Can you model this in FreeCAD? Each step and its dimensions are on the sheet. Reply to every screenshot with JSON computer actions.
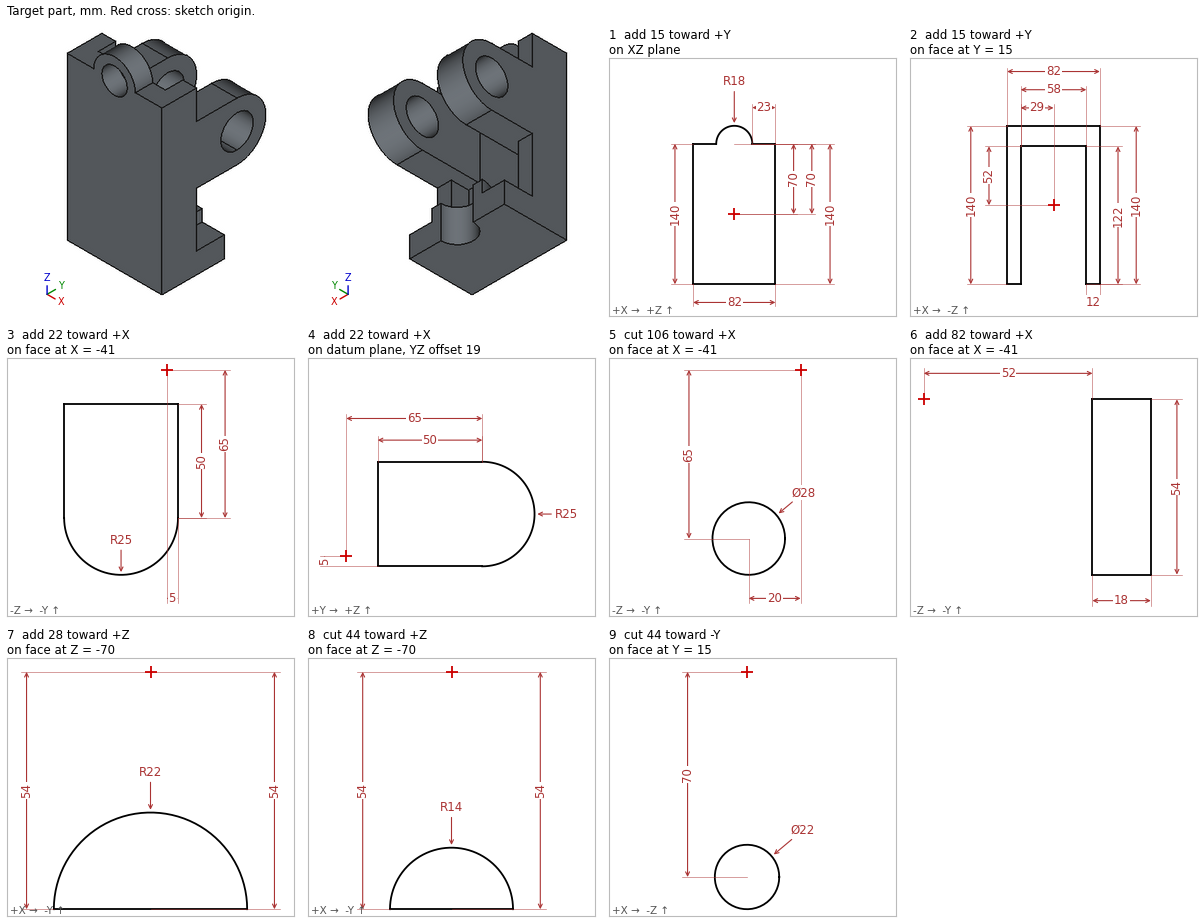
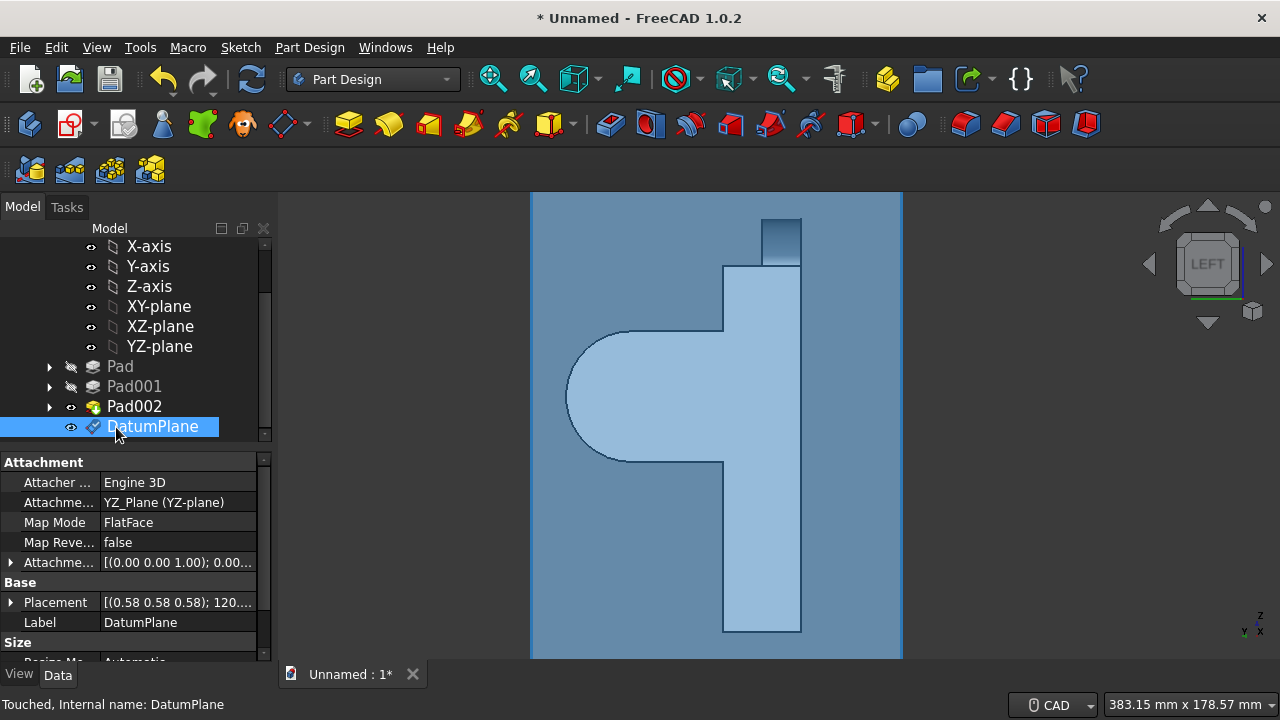
{"action": "left_click", "coordinate": [70, 124]}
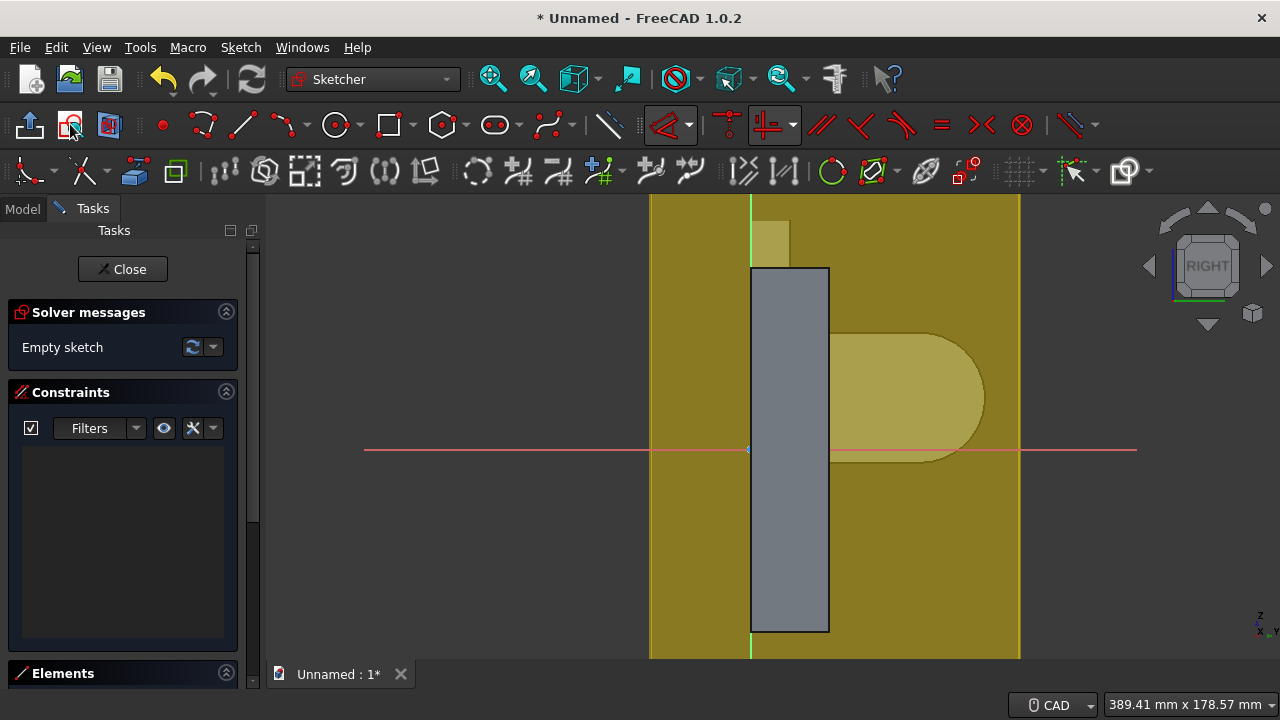
{"action": "key", "text": "q s"}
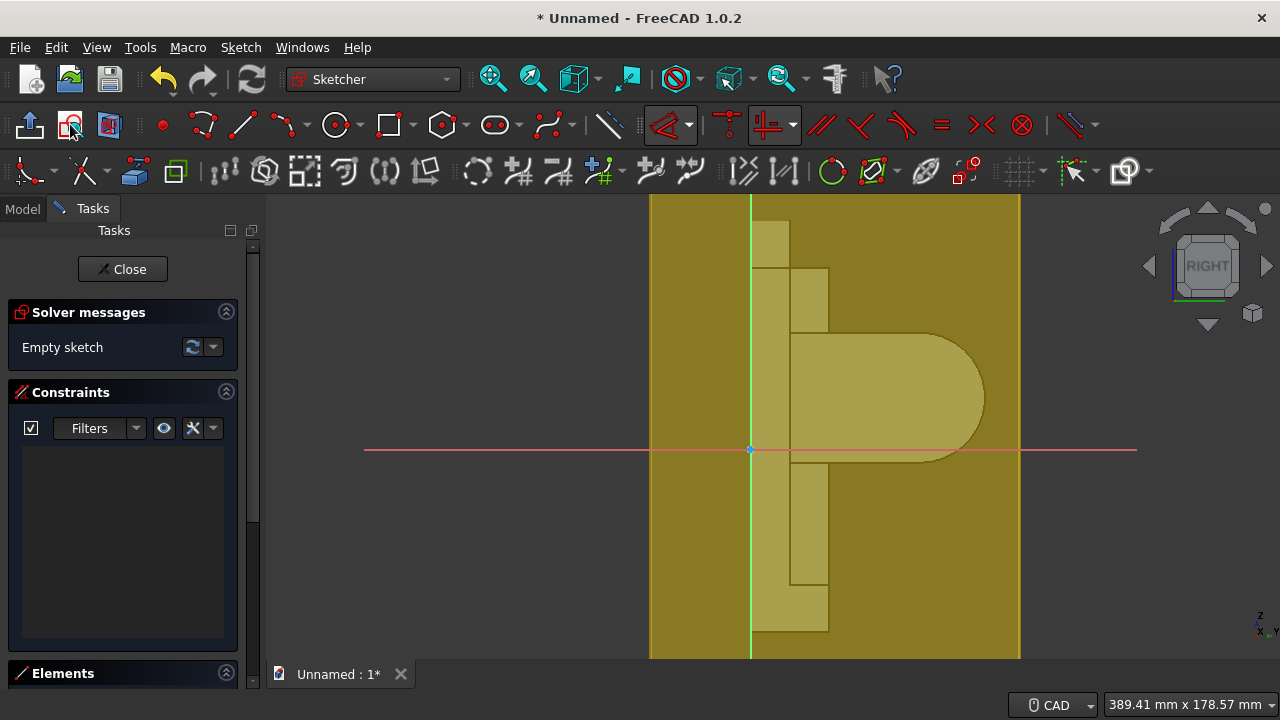
{"action": "scroll", "coordinate": [1001, 374], "scroll_direction": "up", "scroll_amount": 4}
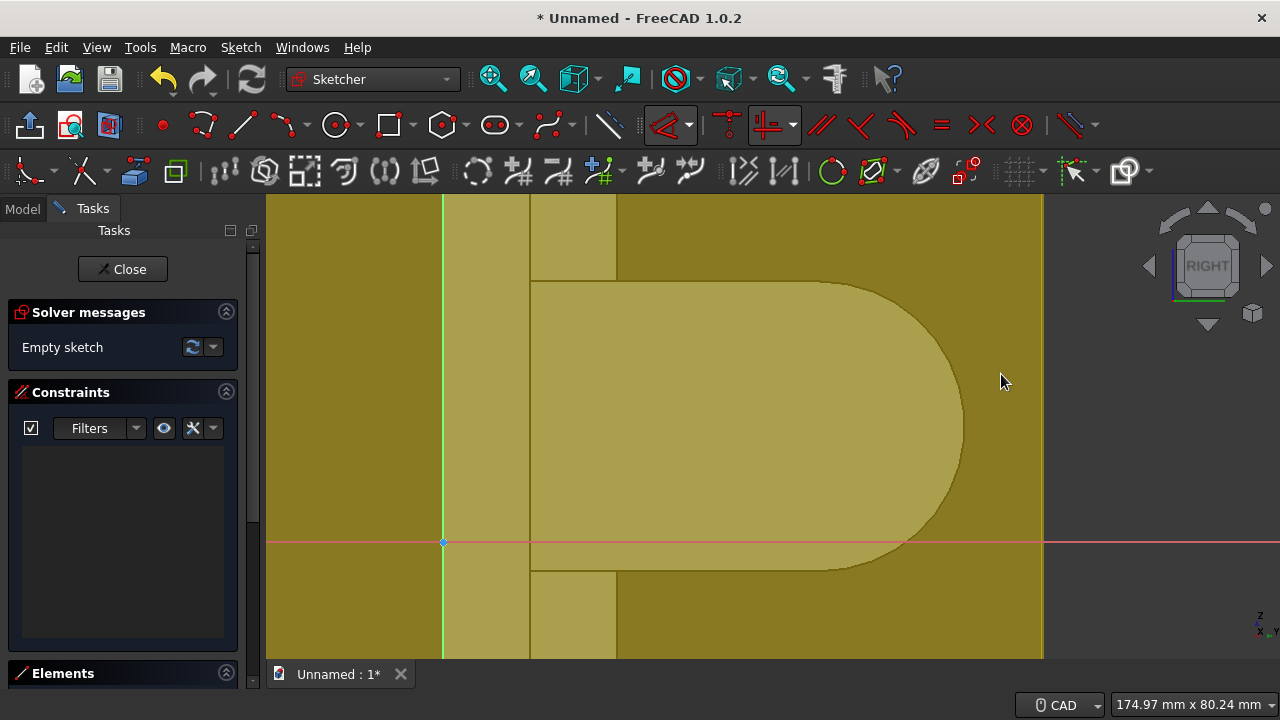
{"action": "key", "text": "g m"}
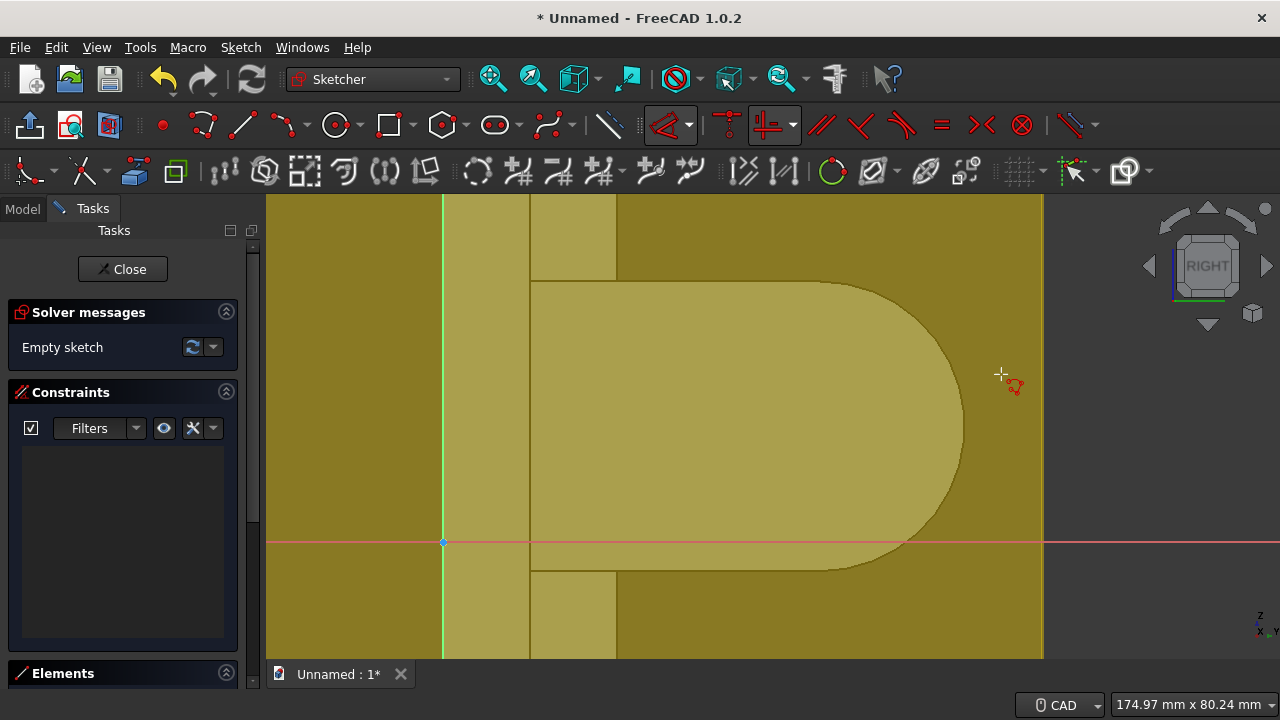
{"action": "left_click", "coordinate": [820, 281]}
{"action": "left_click", "coordinate": [530, 281]}
{"action": "left_click", "coordinate": [530, 571]}
{"action": "left_click", "coordinate": [820, 571]}
{"action": "right_click", "coordinate": [820, 571]}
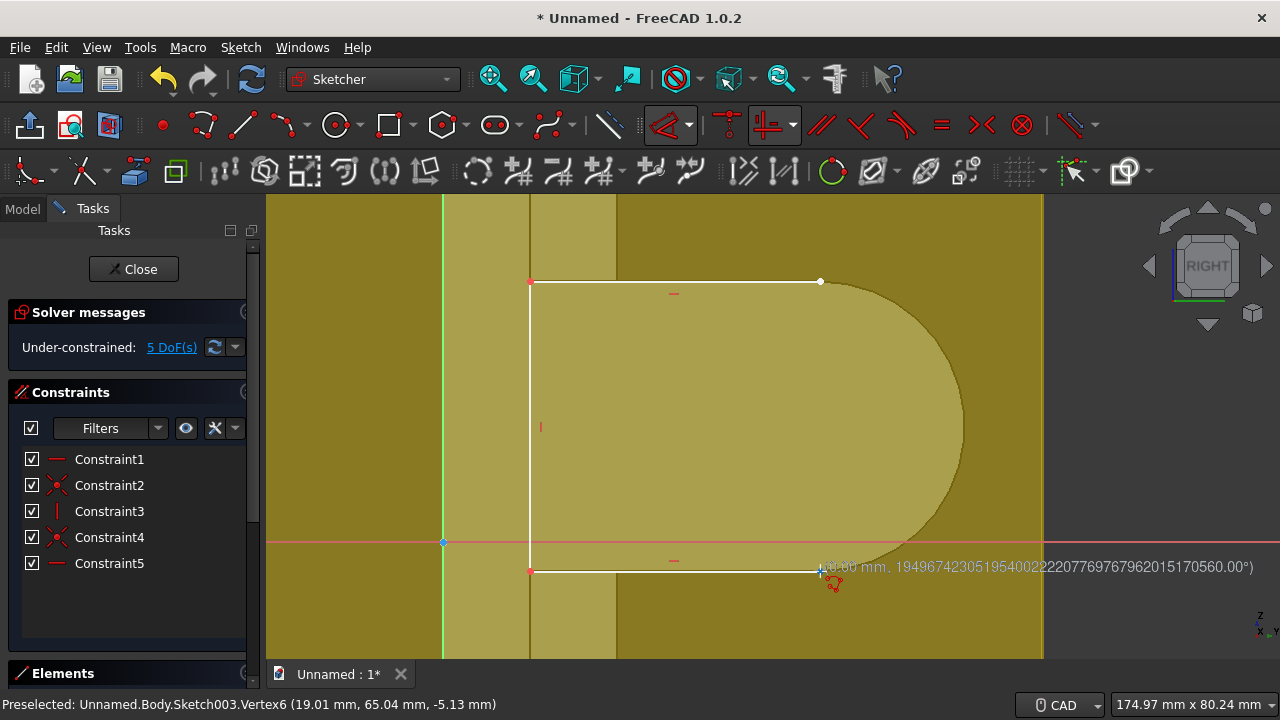
{"action": "left_click", "coordinate": [284, 126]}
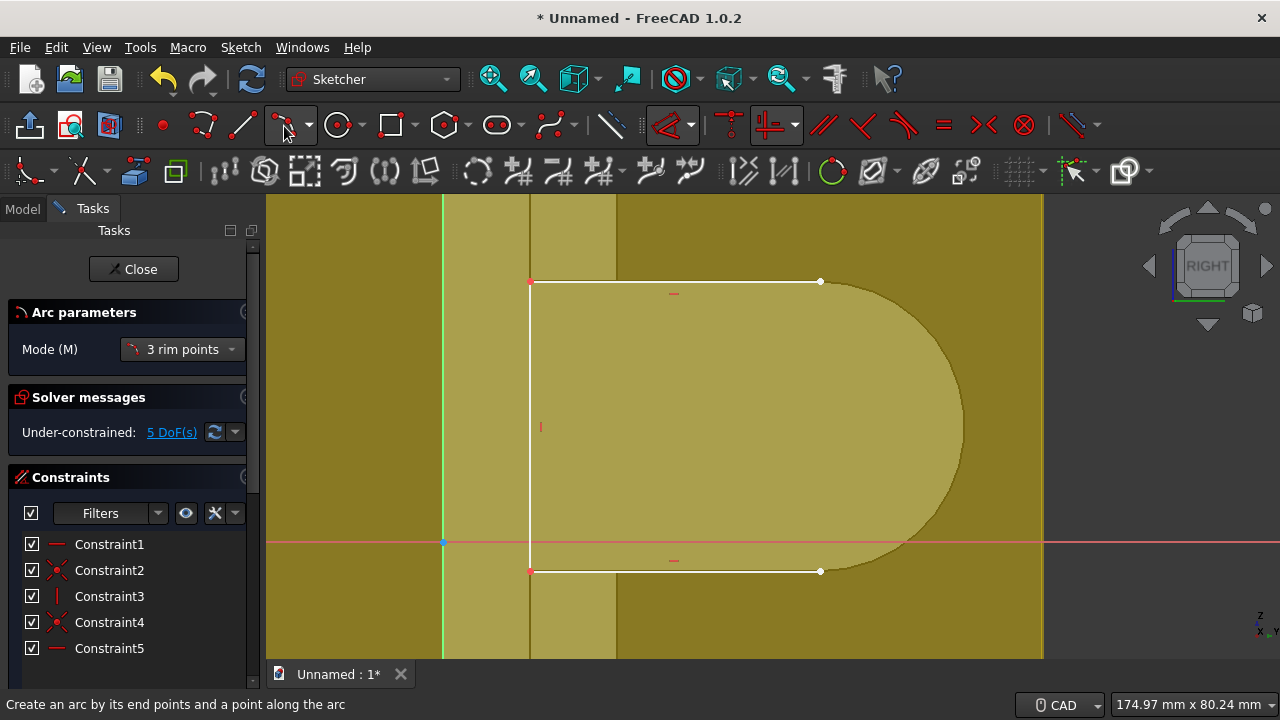
{"action": "left_click", "coordinate": [820, 572]}
{"action": "left_click", "coordinate": [820, 282]}
{"action": "left_click", "coordinate": [965, 426]}
{"action": "key", "text": "Escape"}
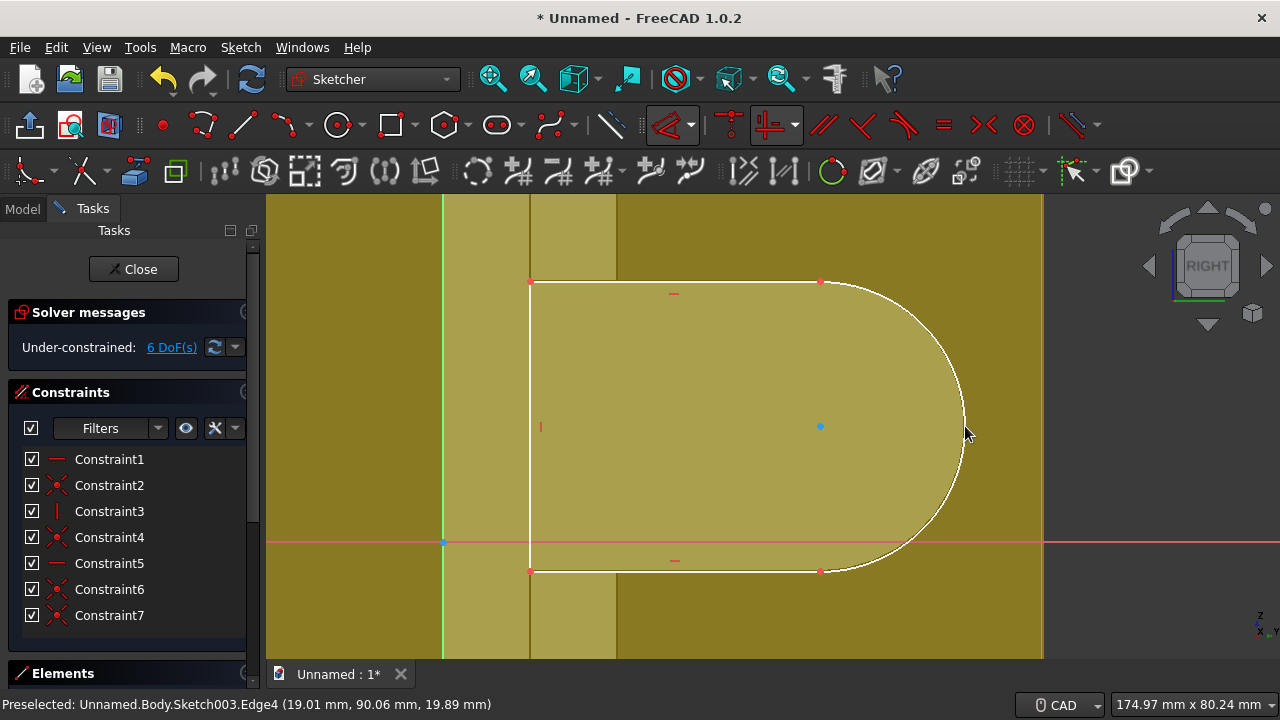
{"action": "left_click", "coordinate": [733, 282]}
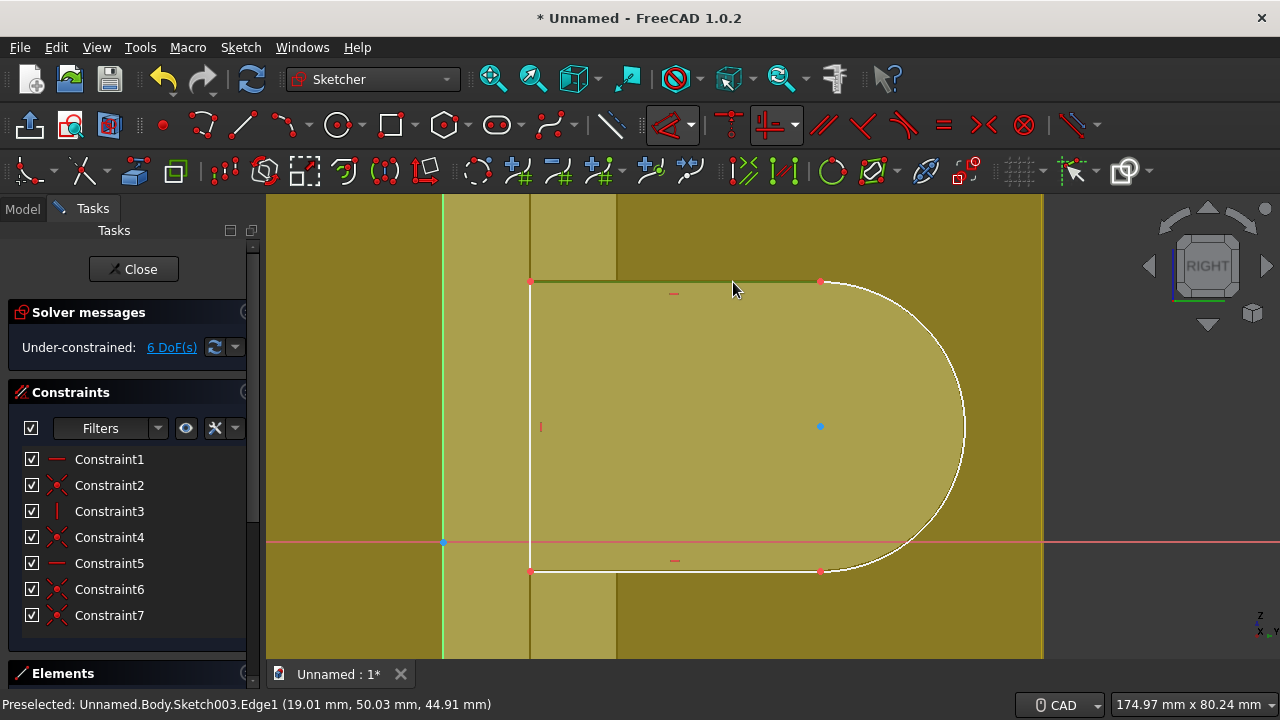
{"action": "left_click", "coordinate": [937, 512]}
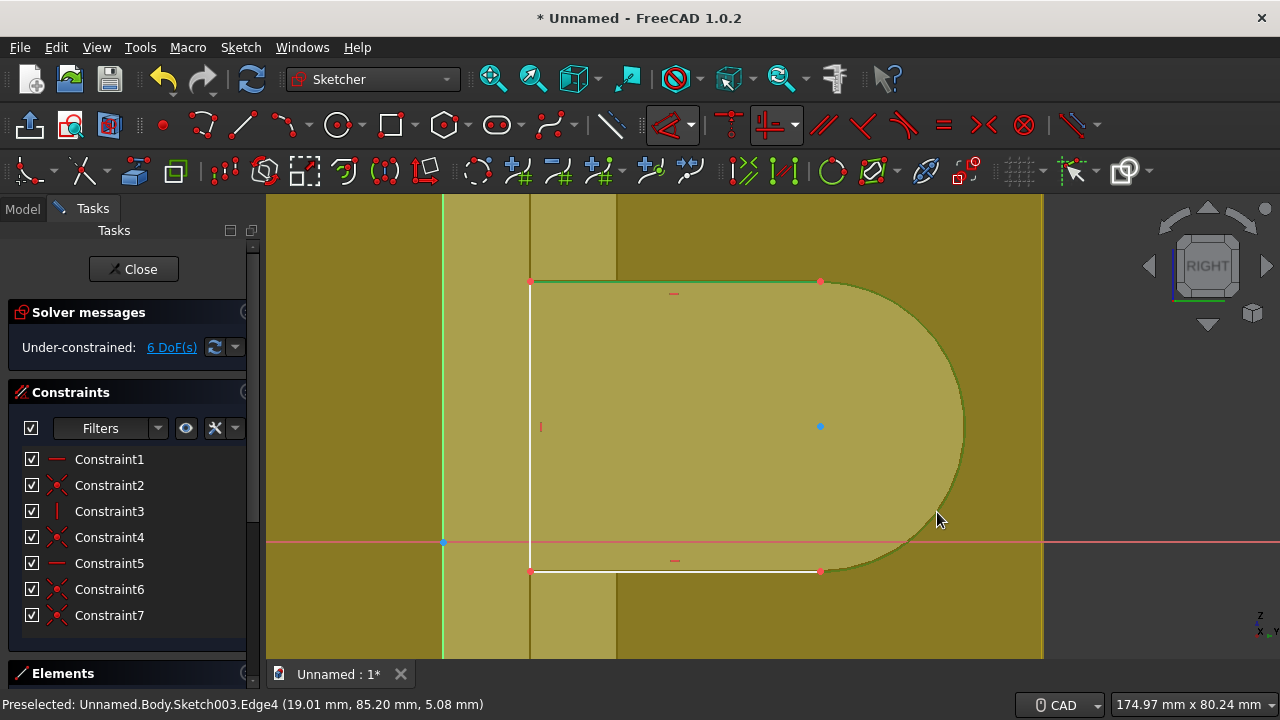
{"action": "key", "text": "t"}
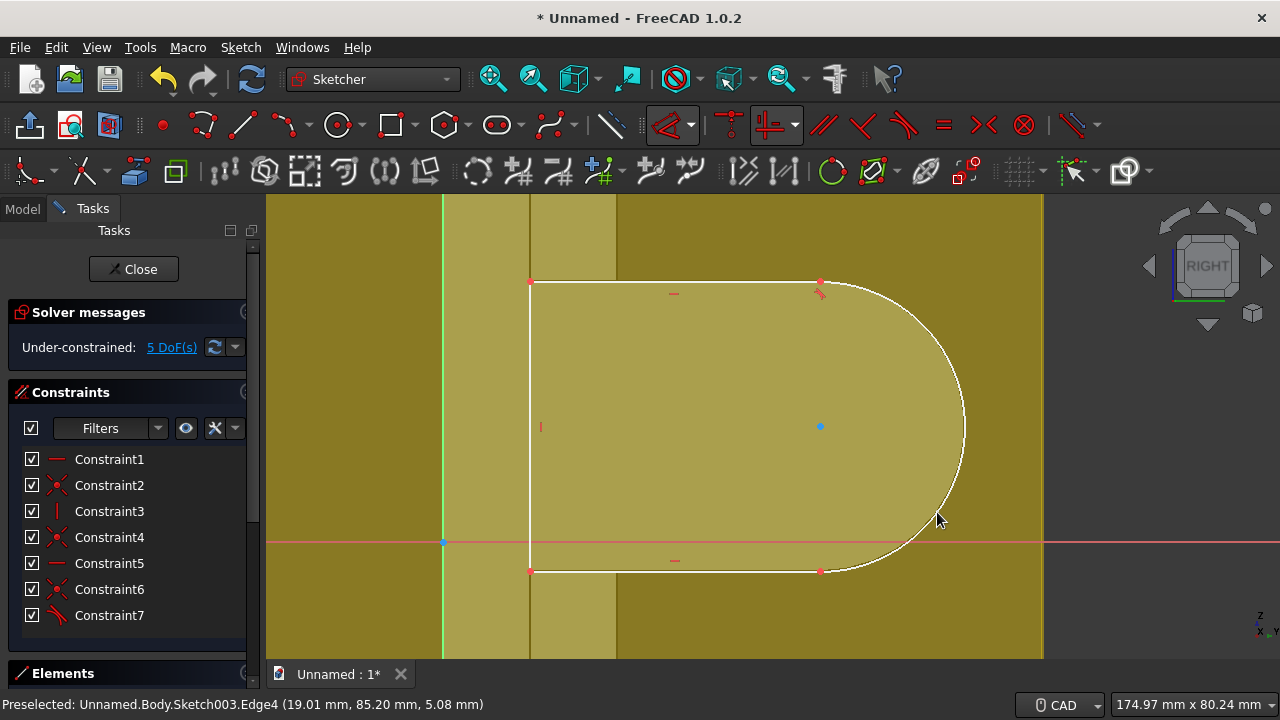
{"action": "left_click", "coordinate": [617, 572]}